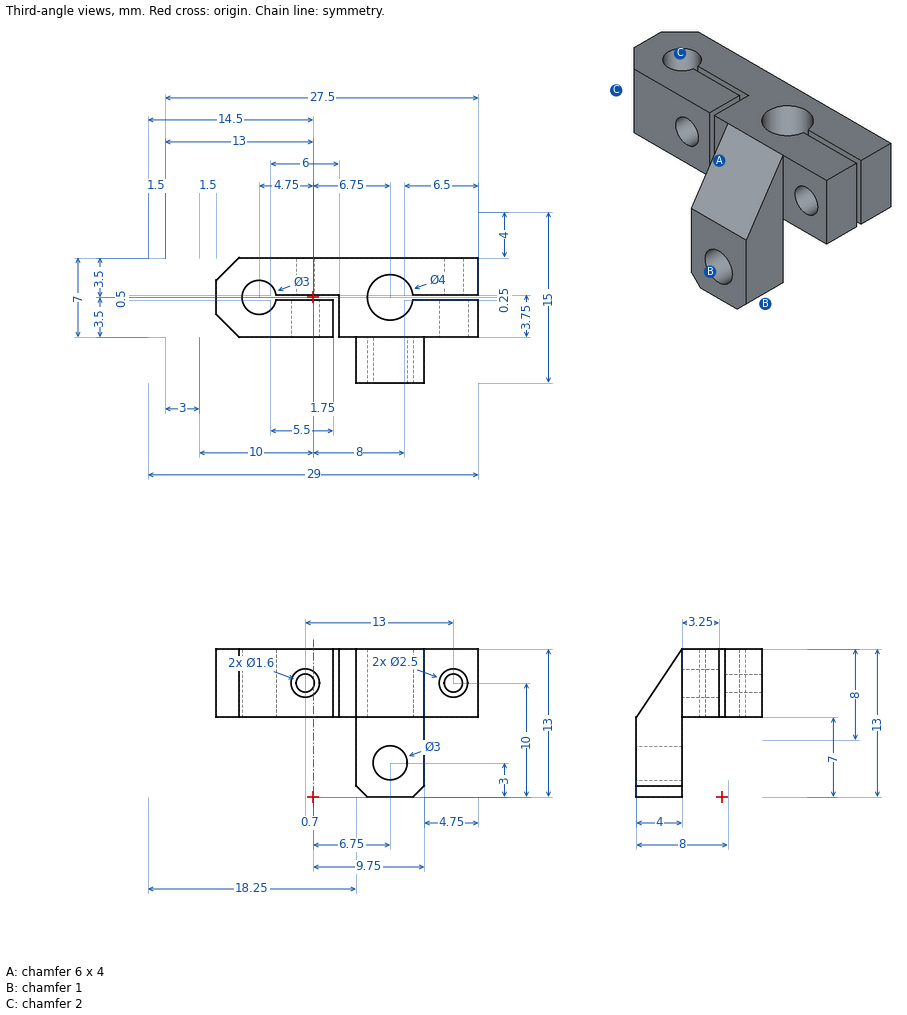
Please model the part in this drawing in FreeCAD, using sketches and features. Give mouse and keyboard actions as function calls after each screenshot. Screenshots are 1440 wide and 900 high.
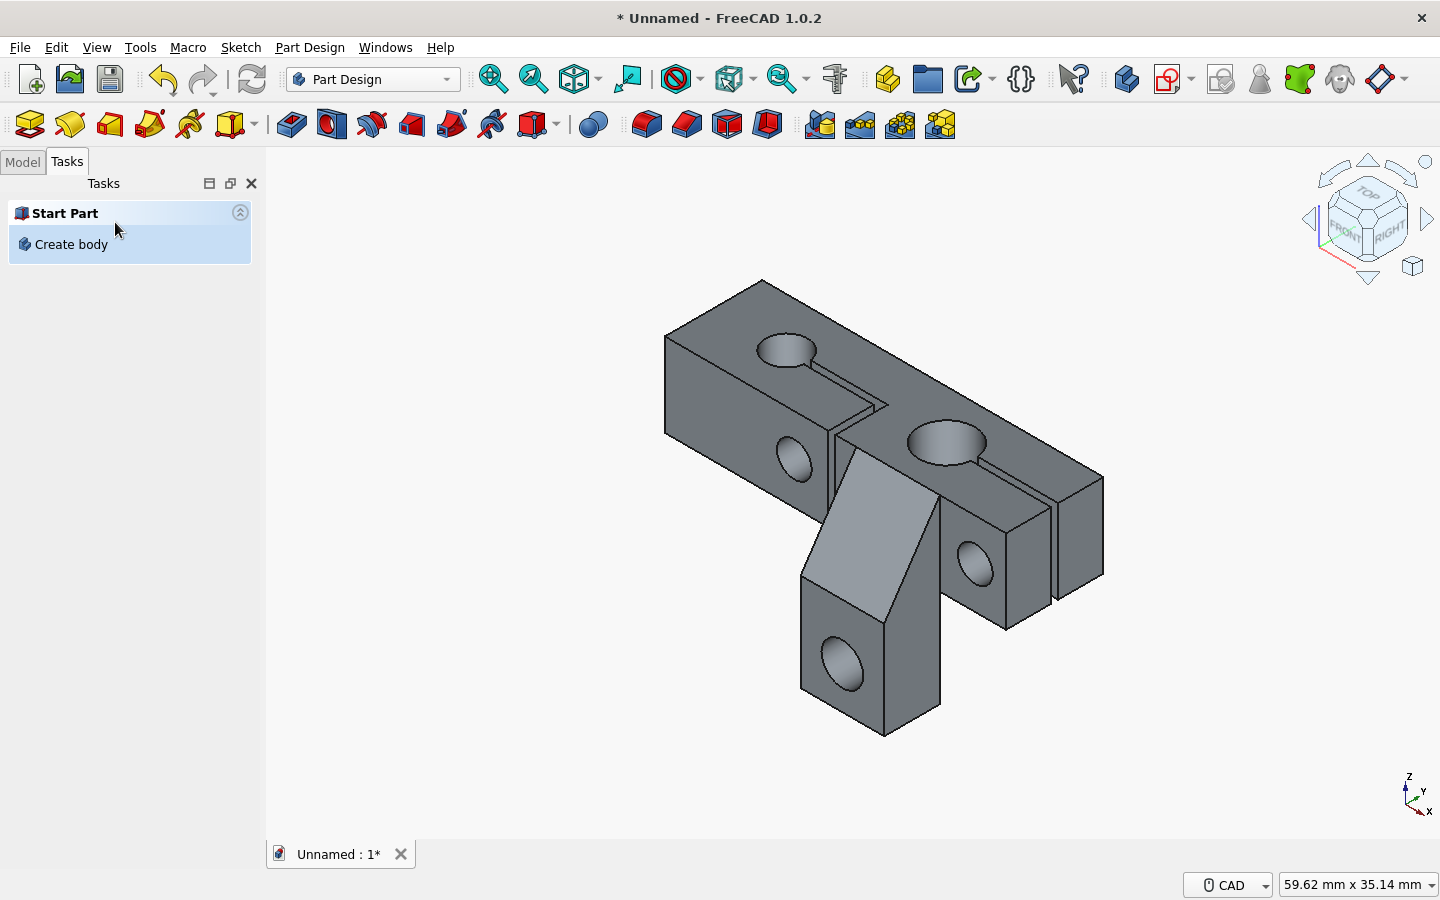
key(2)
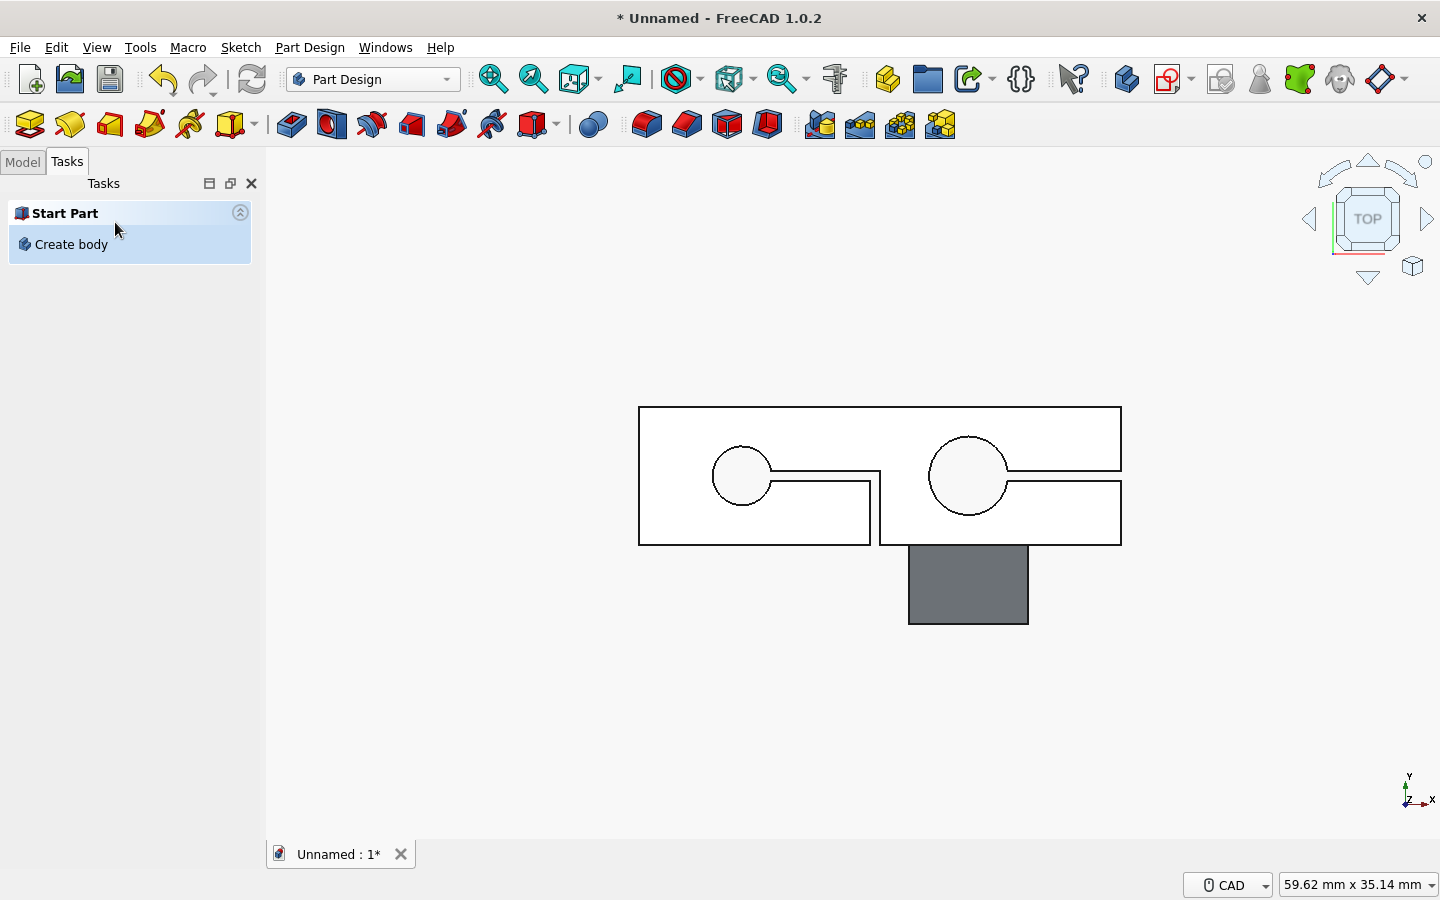
click(494, 80)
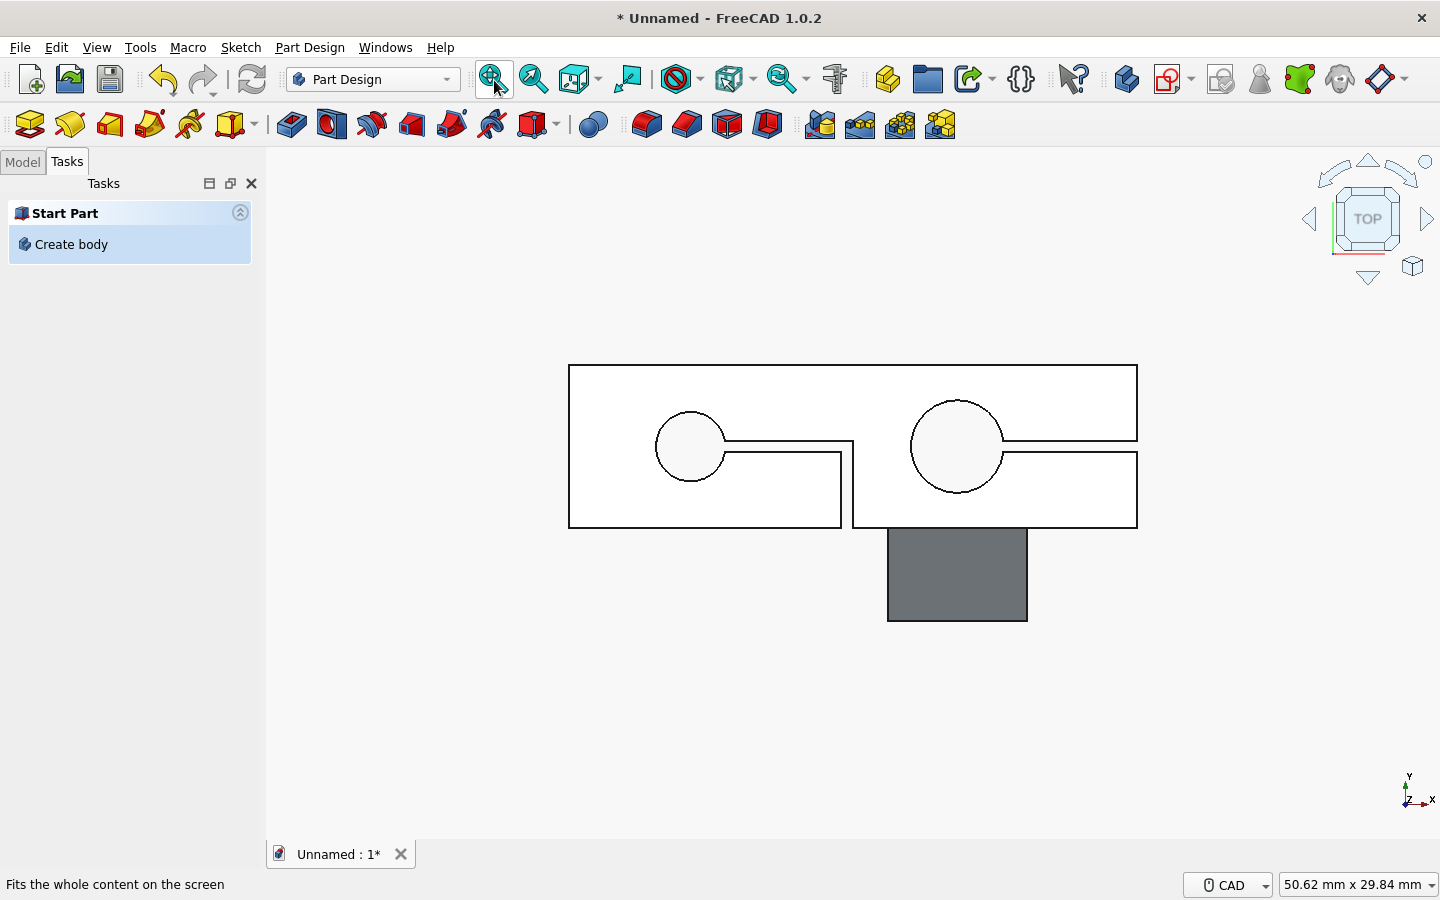
key(0)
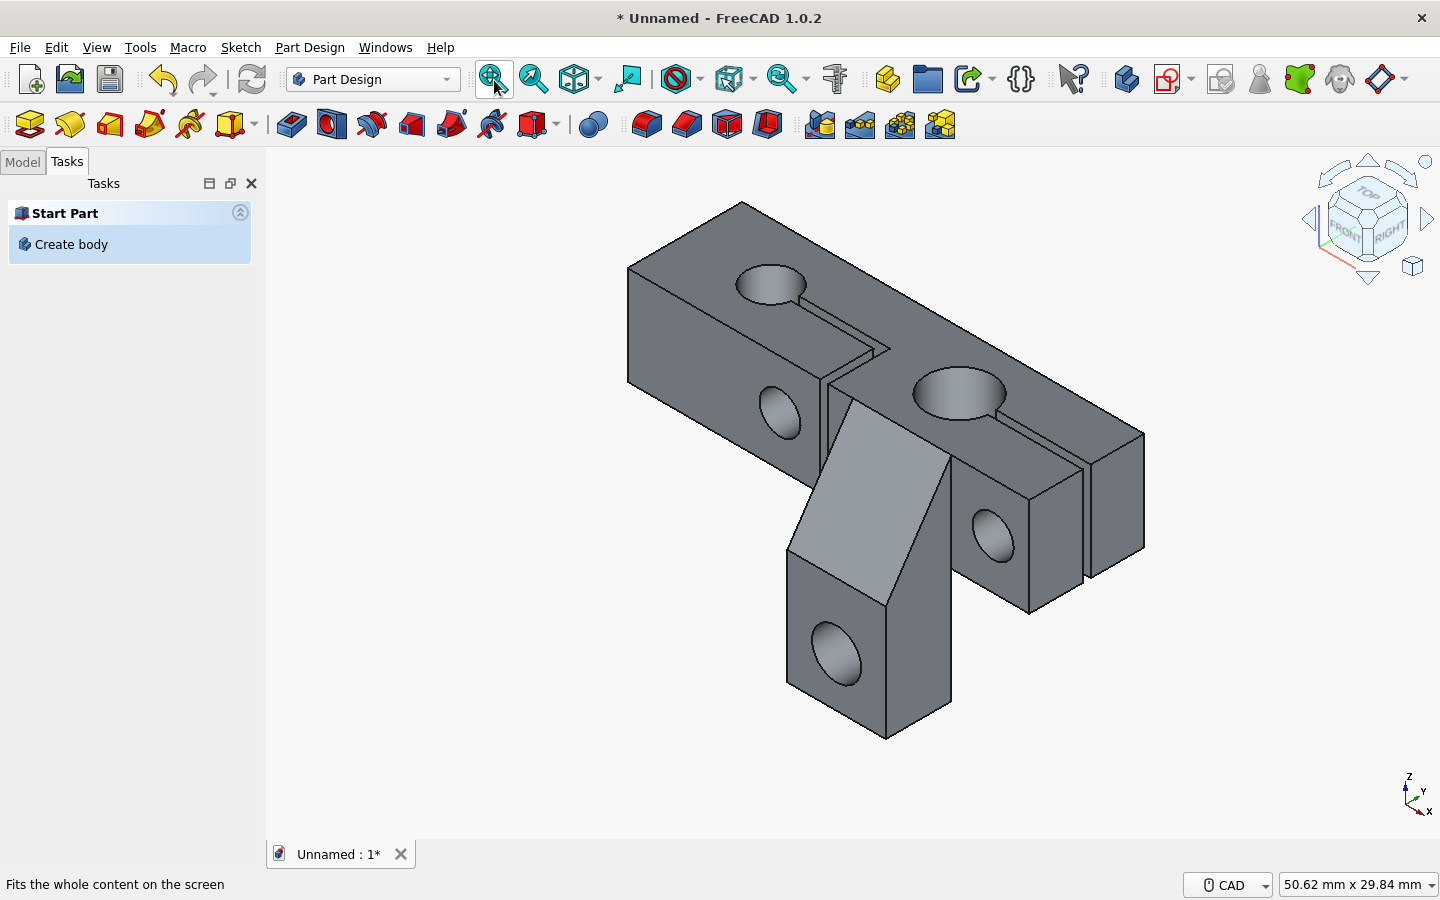
key(1)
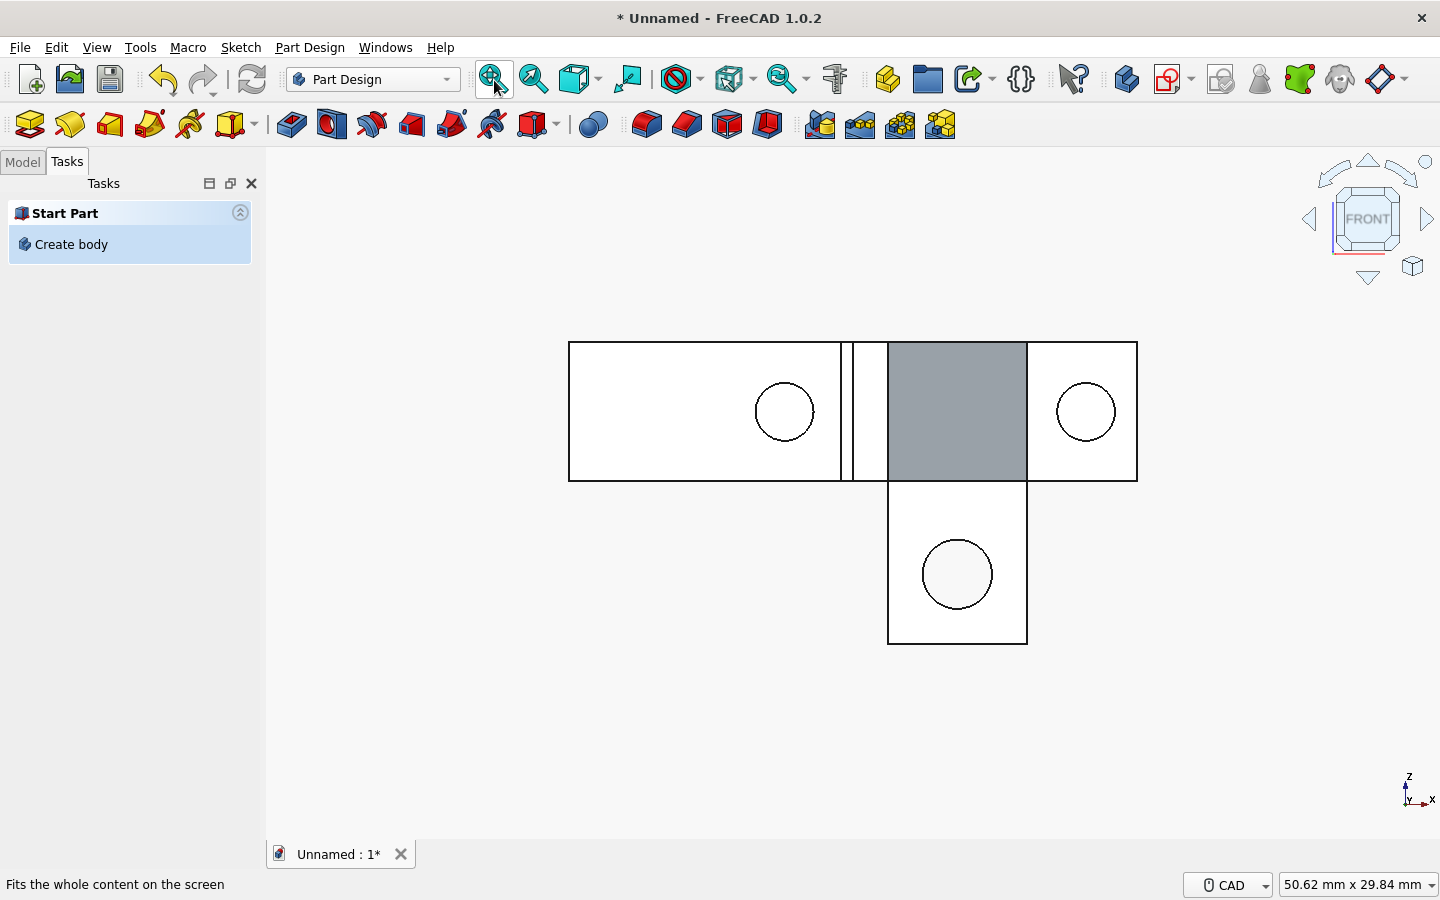
key(3)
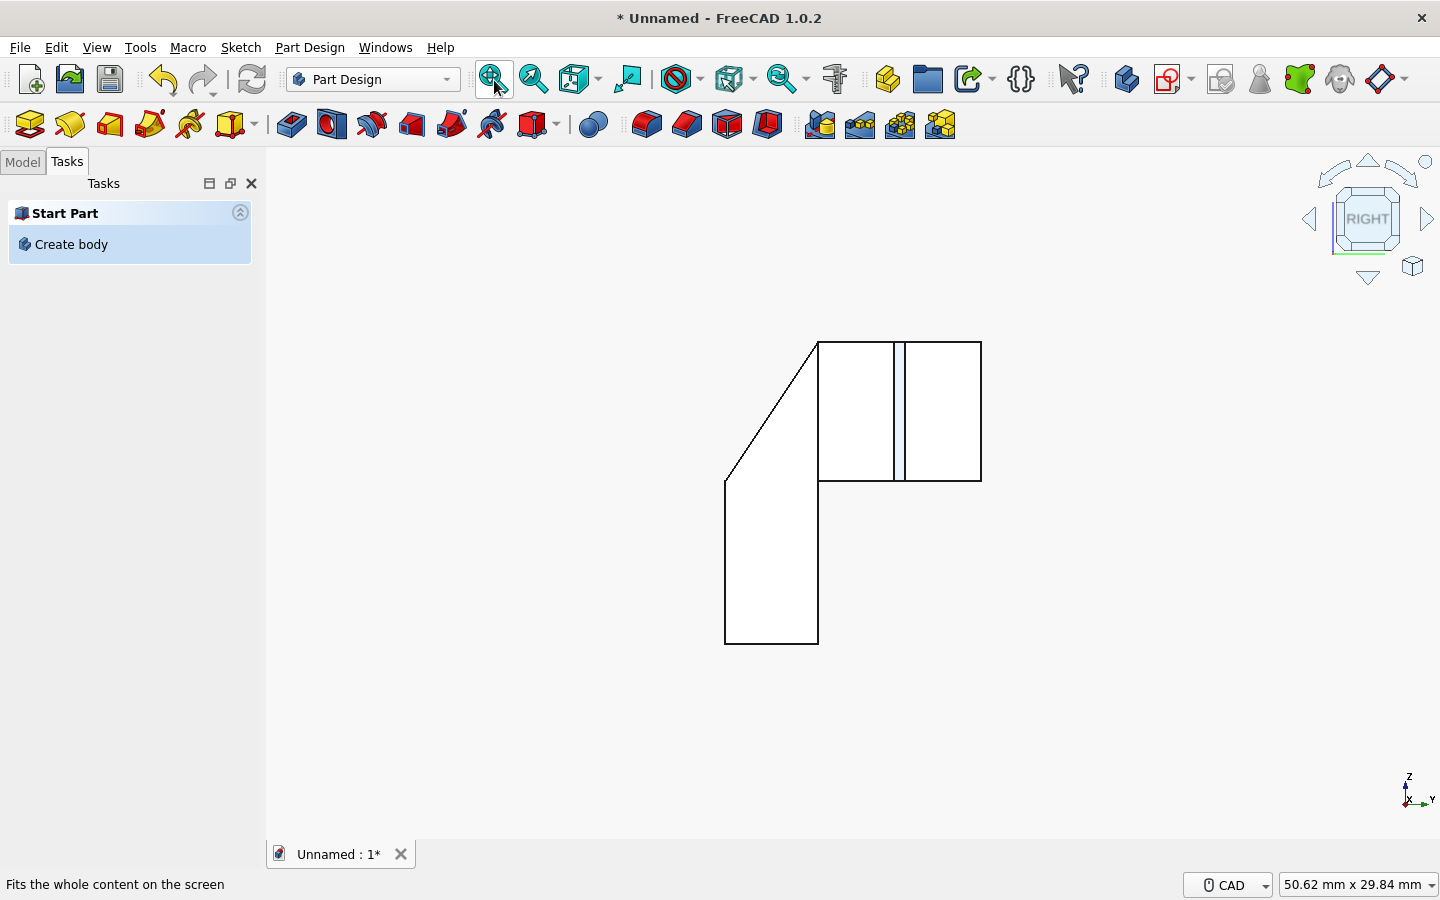
click(494, 80)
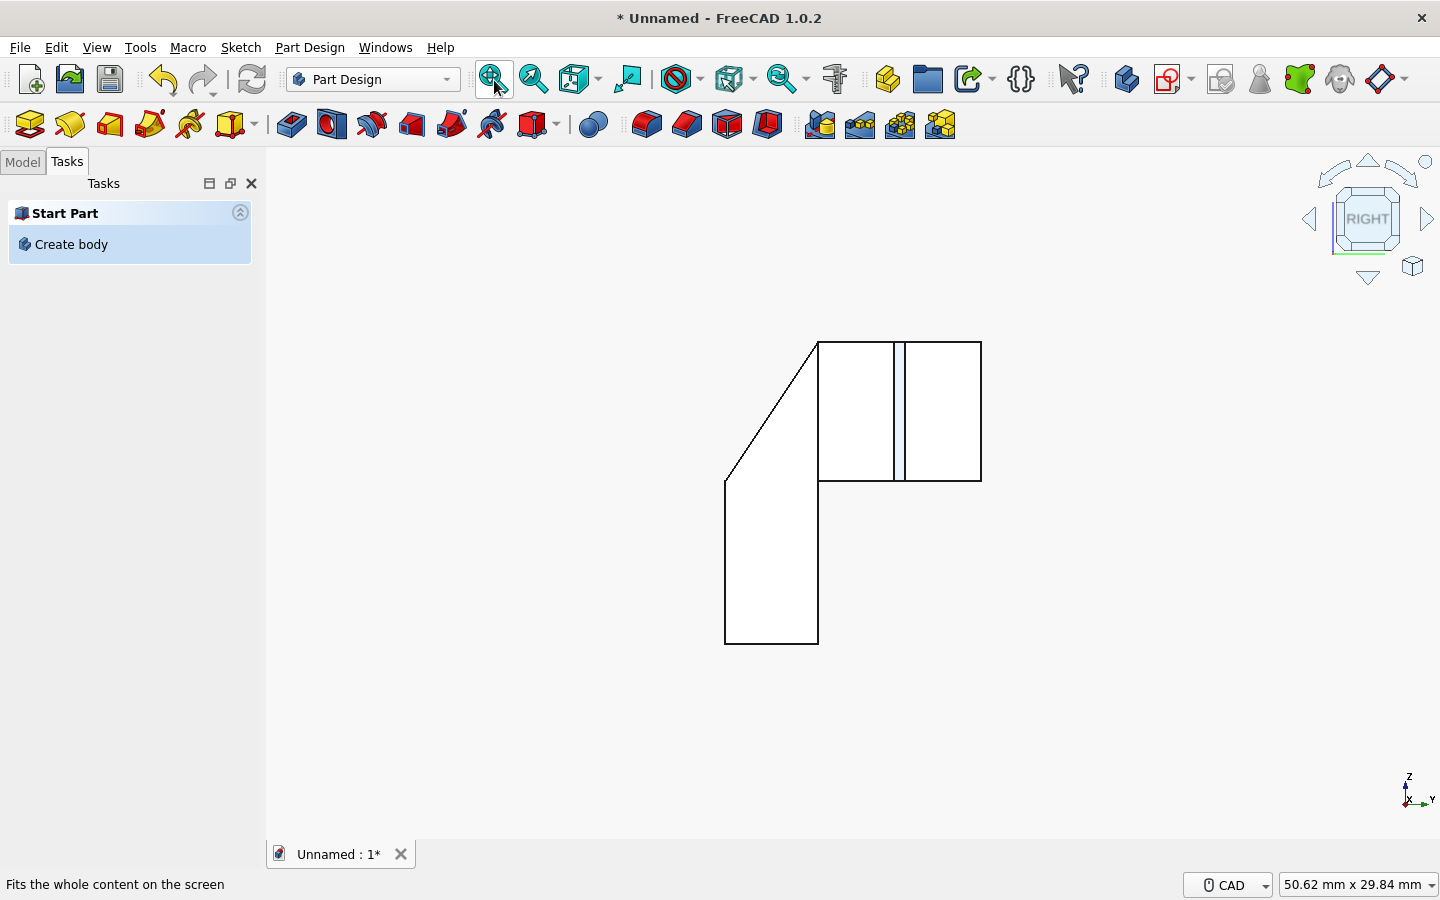
click(772, 643)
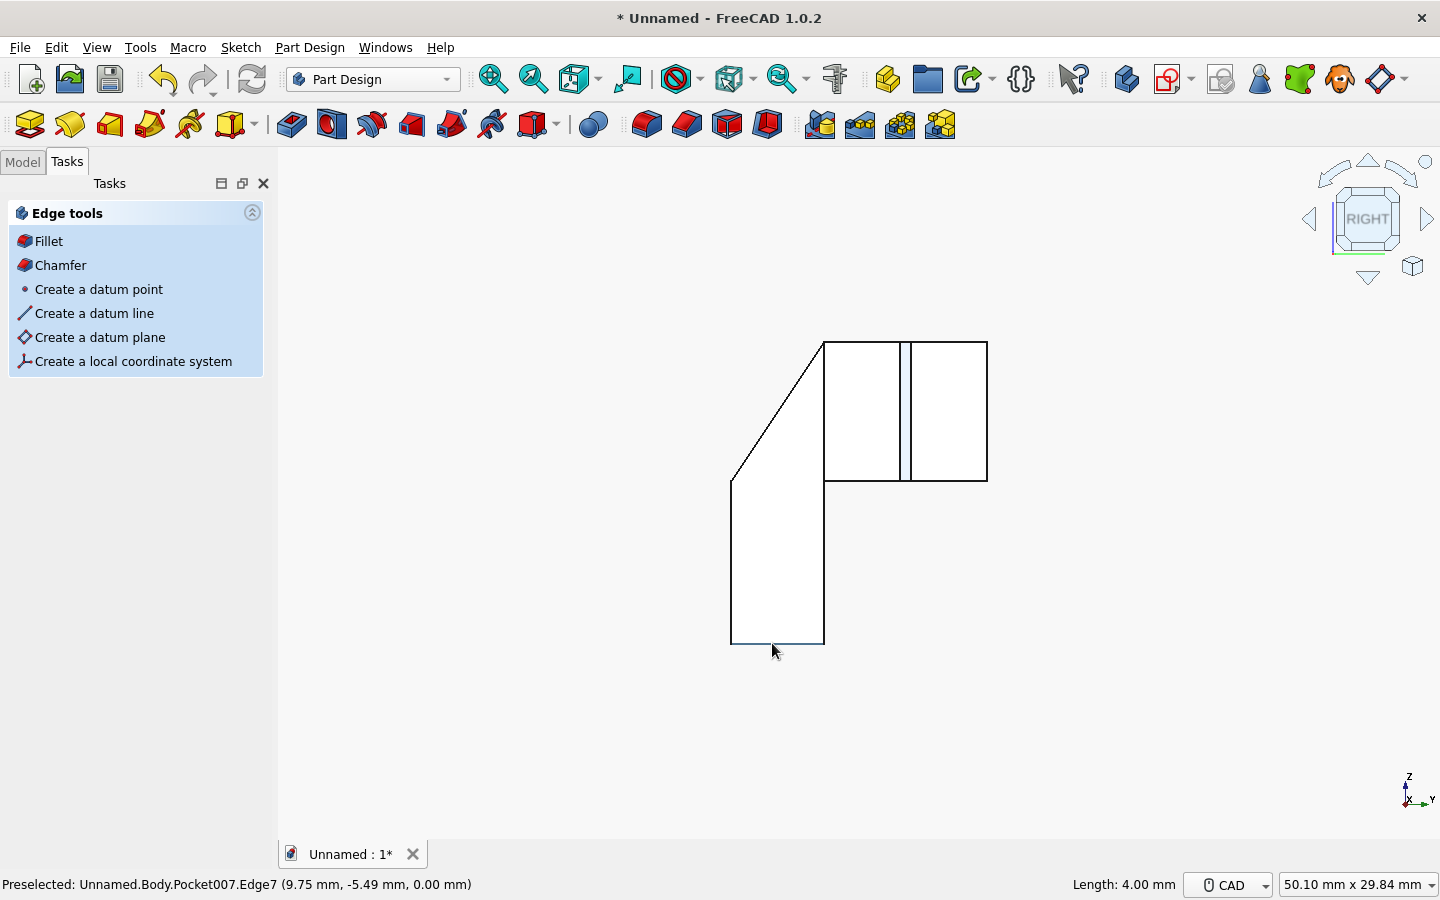
key(5)